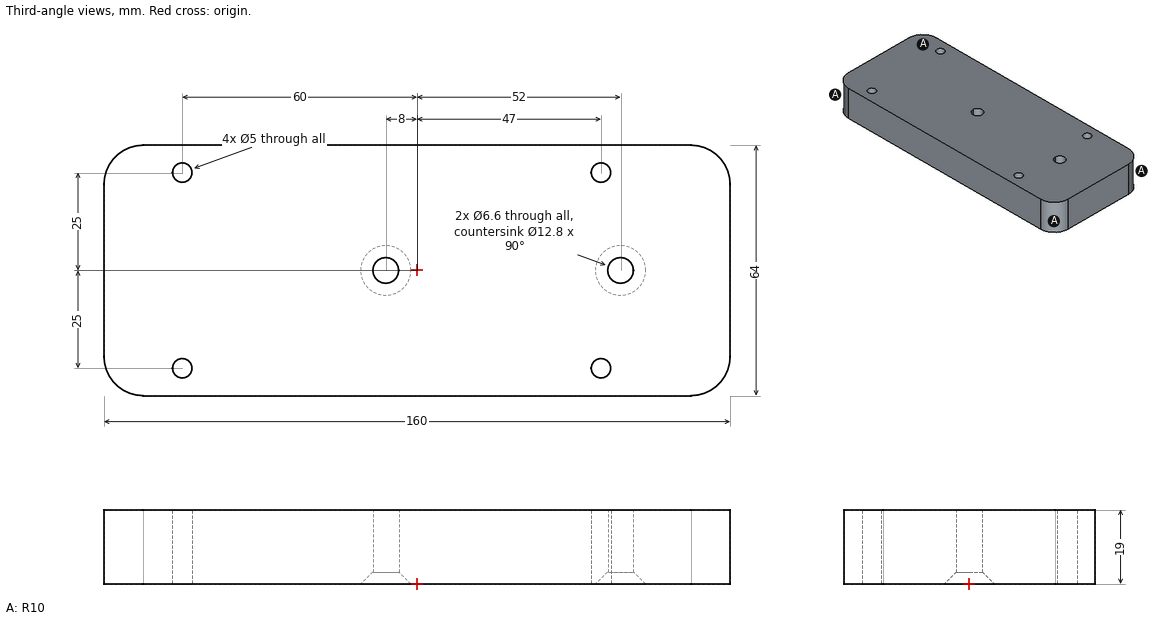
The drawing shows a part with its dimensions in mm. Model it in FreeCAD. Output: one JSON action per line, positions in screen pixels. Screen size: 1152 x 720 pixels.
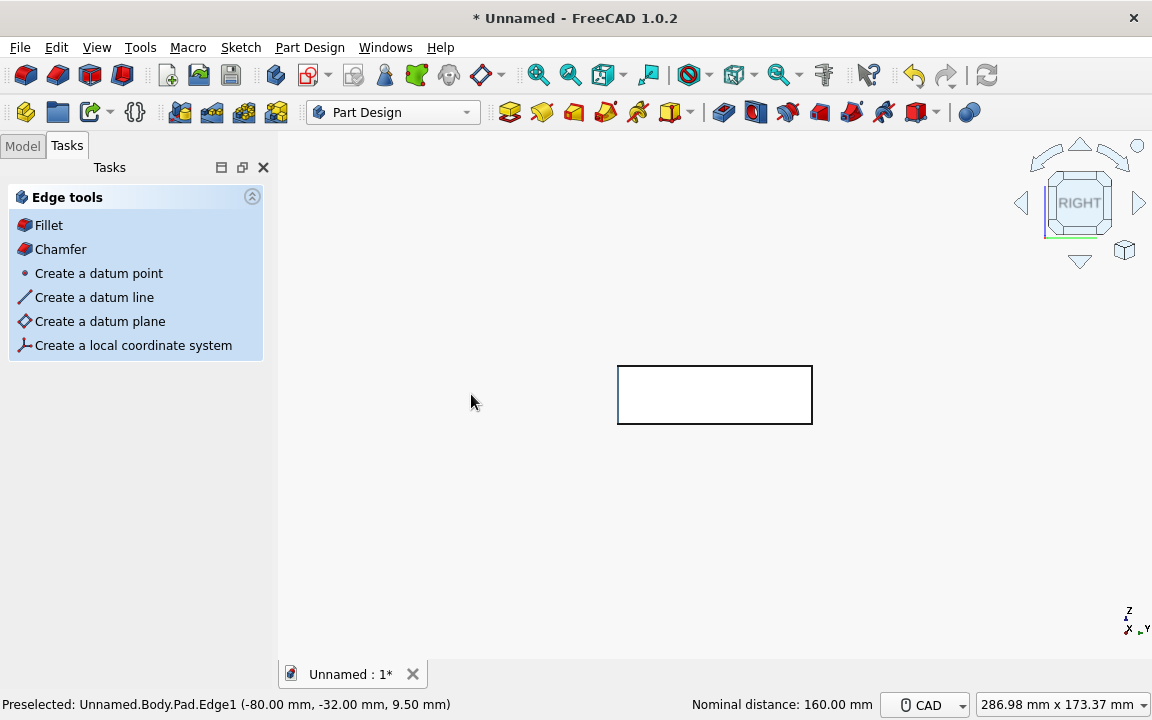
{"action": "left_click", "coordinate": [540, 76]}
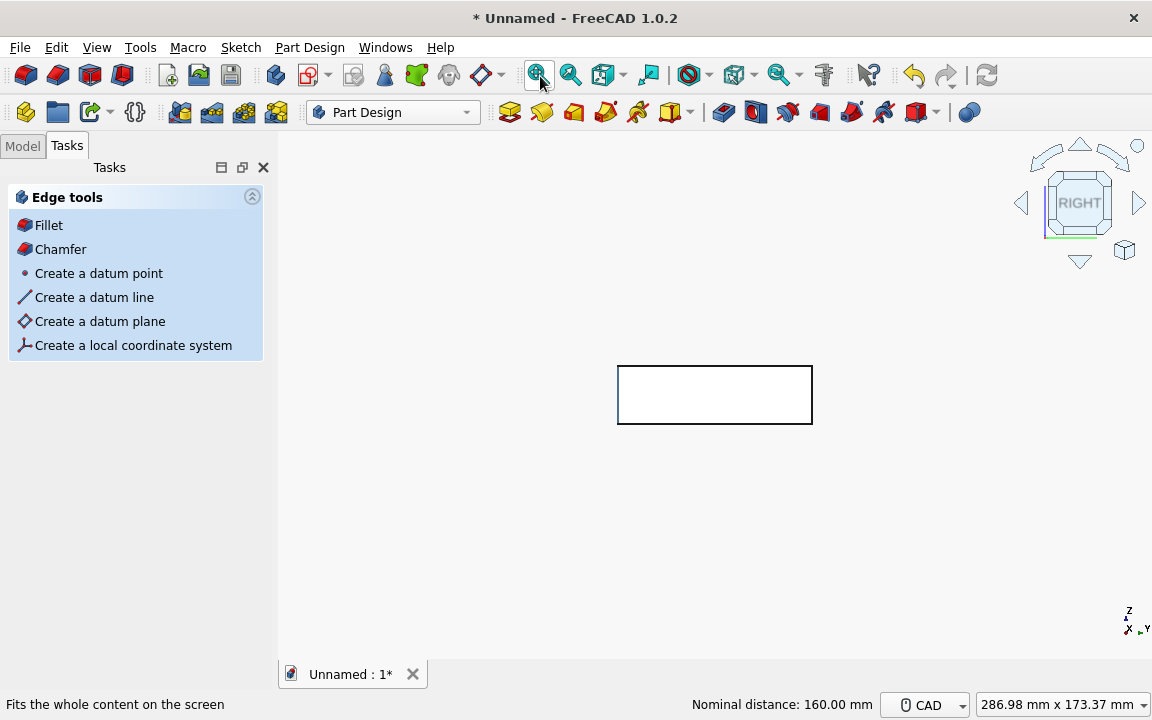
{"action": "left_click", "coordinate": [812, 394], "text": "ctrl"}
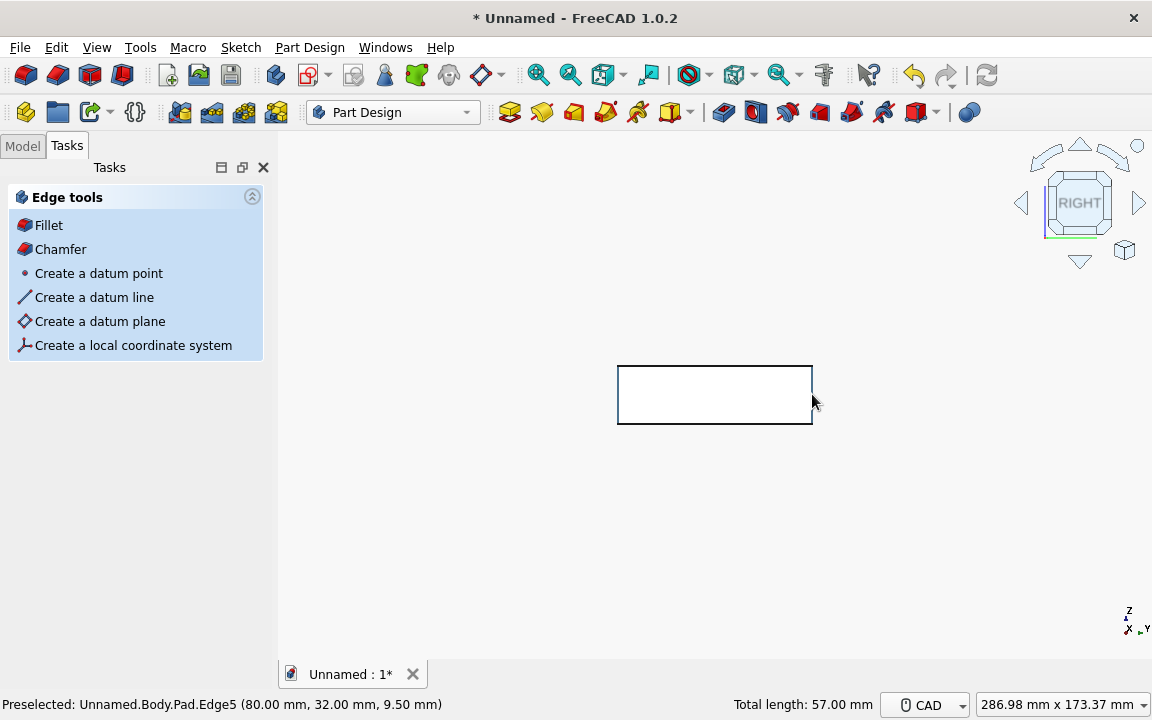
{"action": "key", "text": "5"}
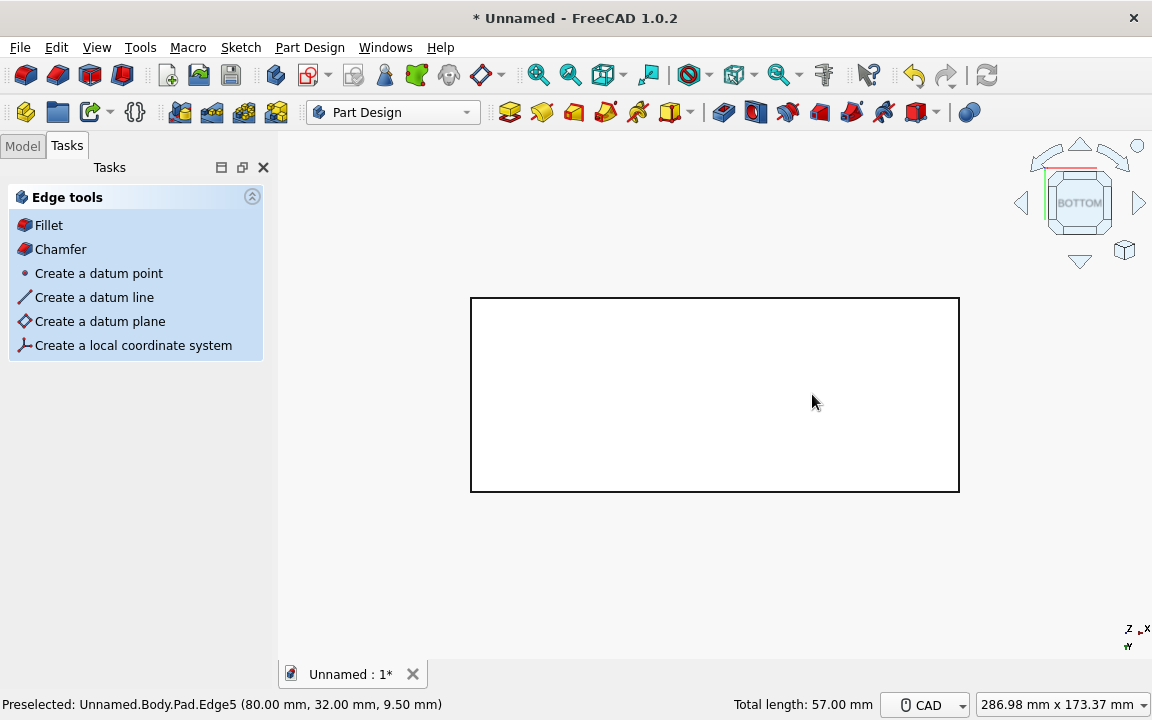
{"action": "key", "text": "4"}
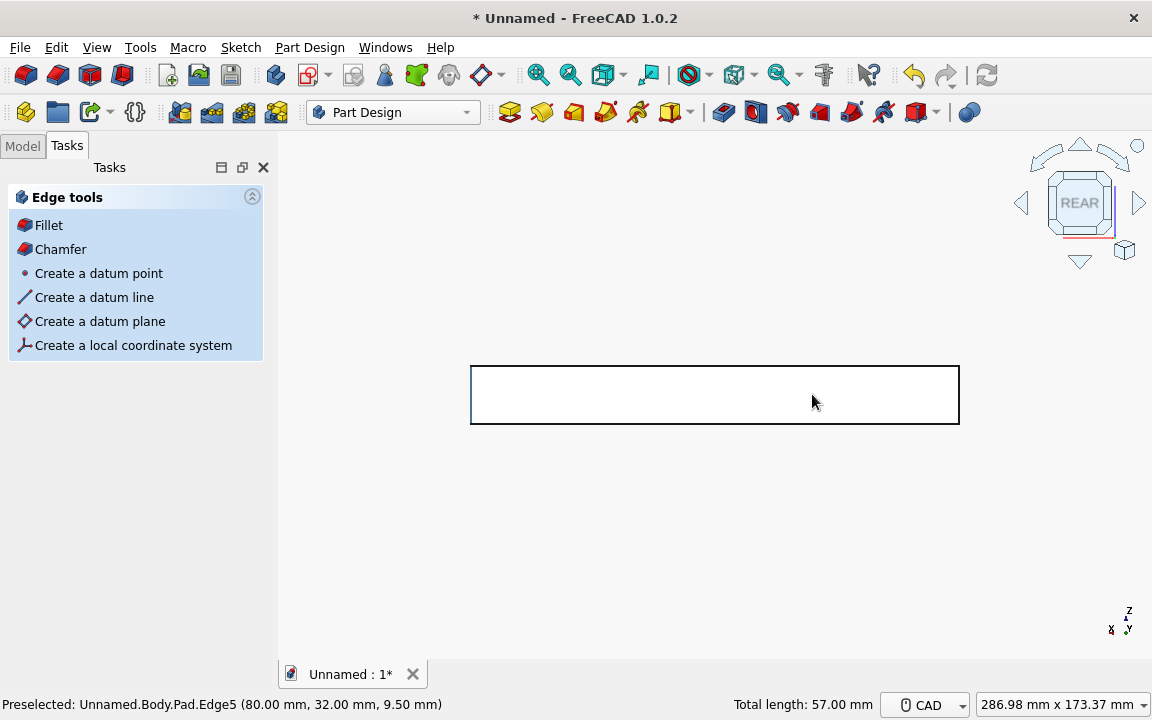
{"action": "left_click", "coordinate": [959, 394], "text": "ctrl"}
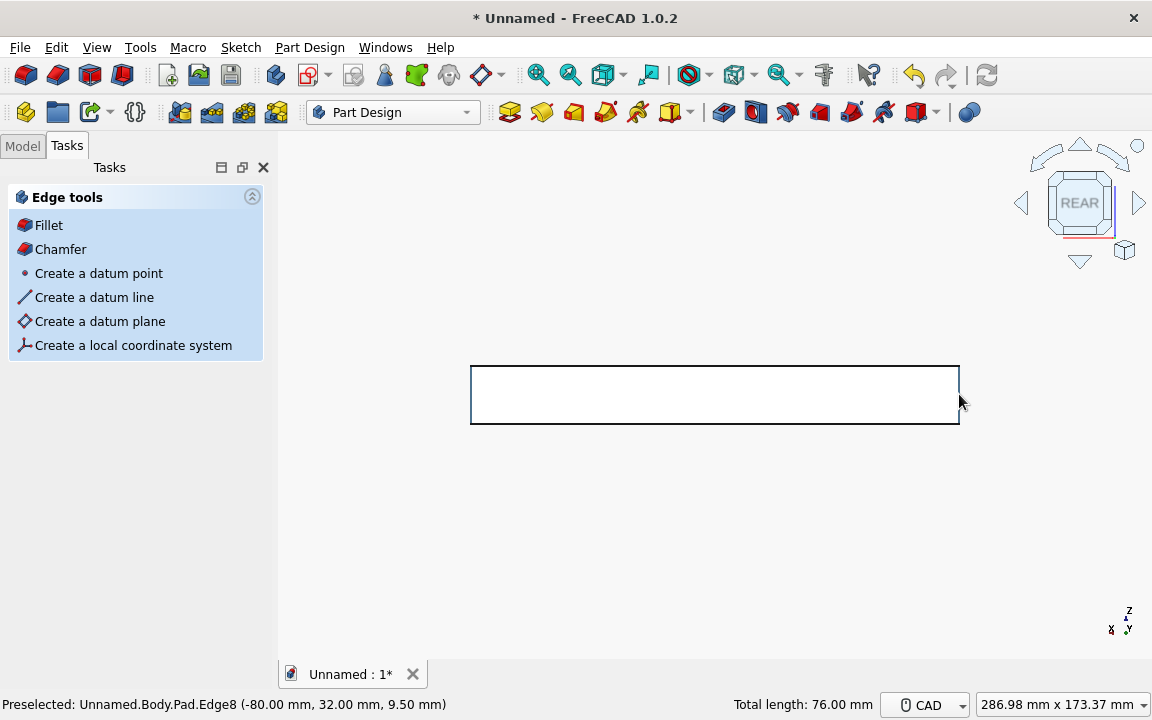
{"action": "left_click", "coordinate": [26, 76]}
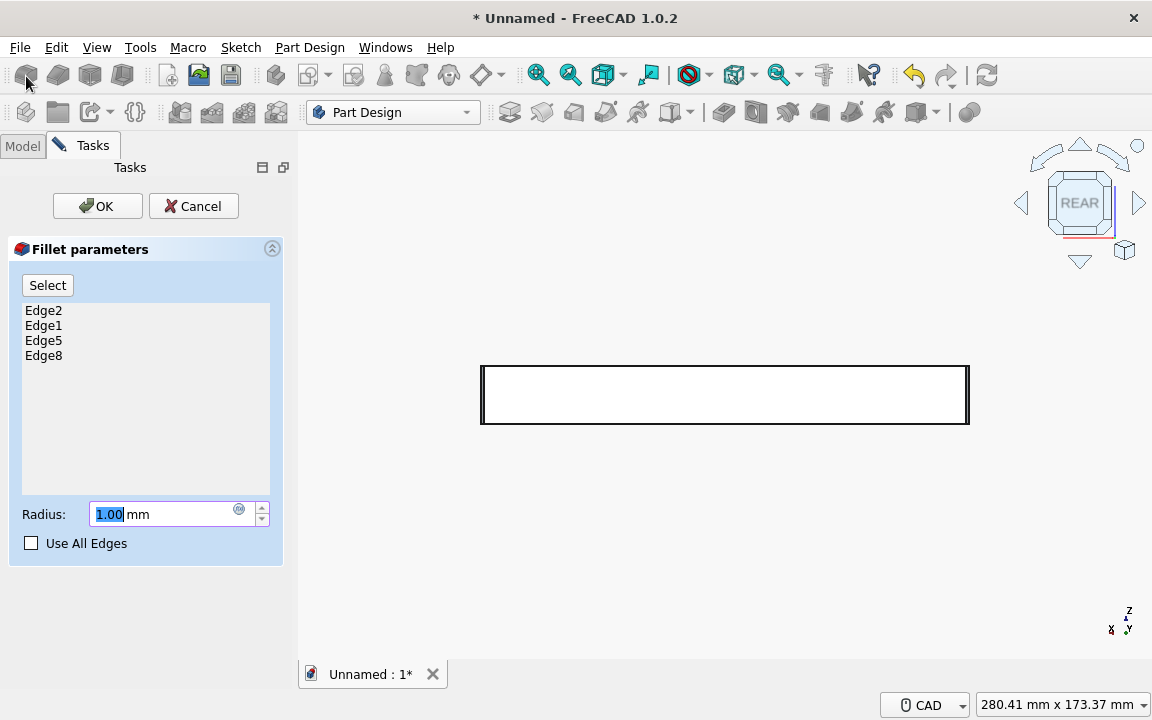
{"action": "type", "text": "10"}
{"action": "key", "text": "Tab"}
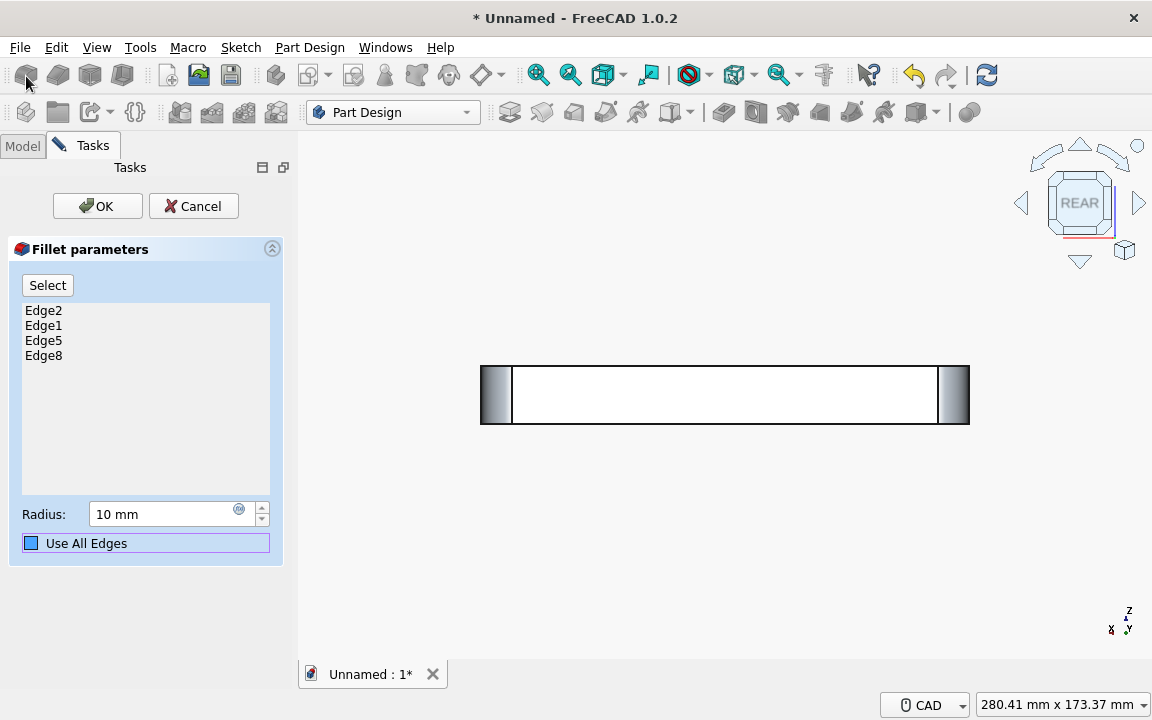
{"action": "left_click", "coordinate": [98, 206]}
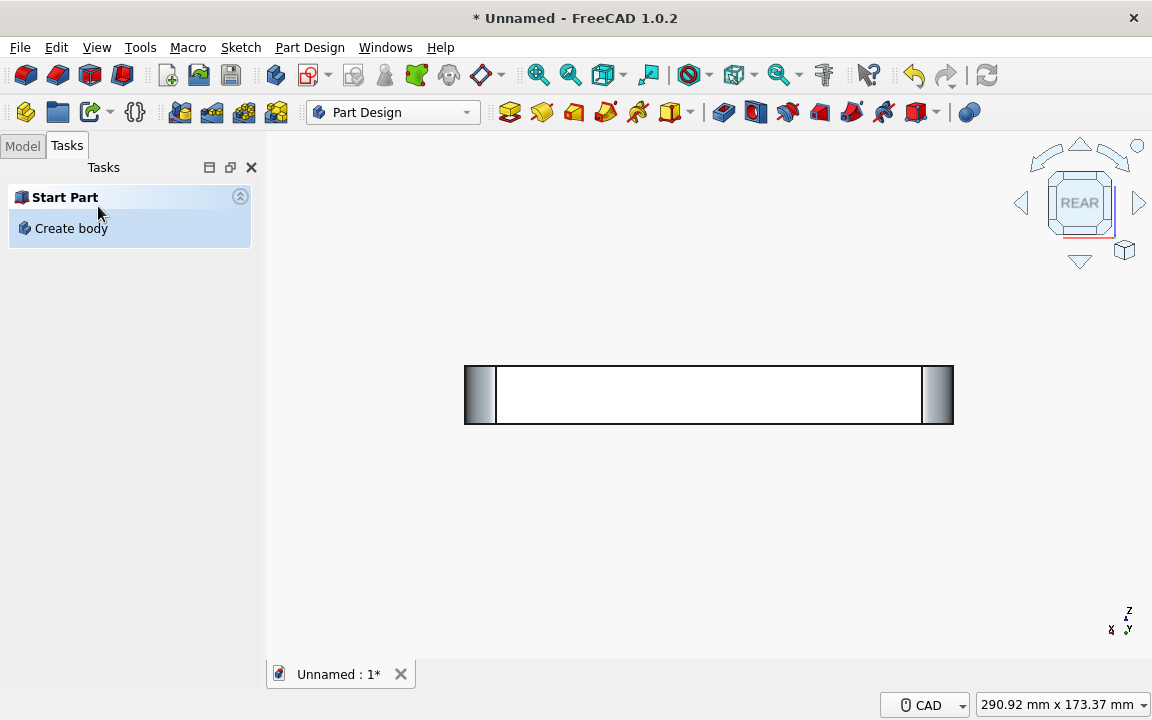
{"action": "key", "text": "0"}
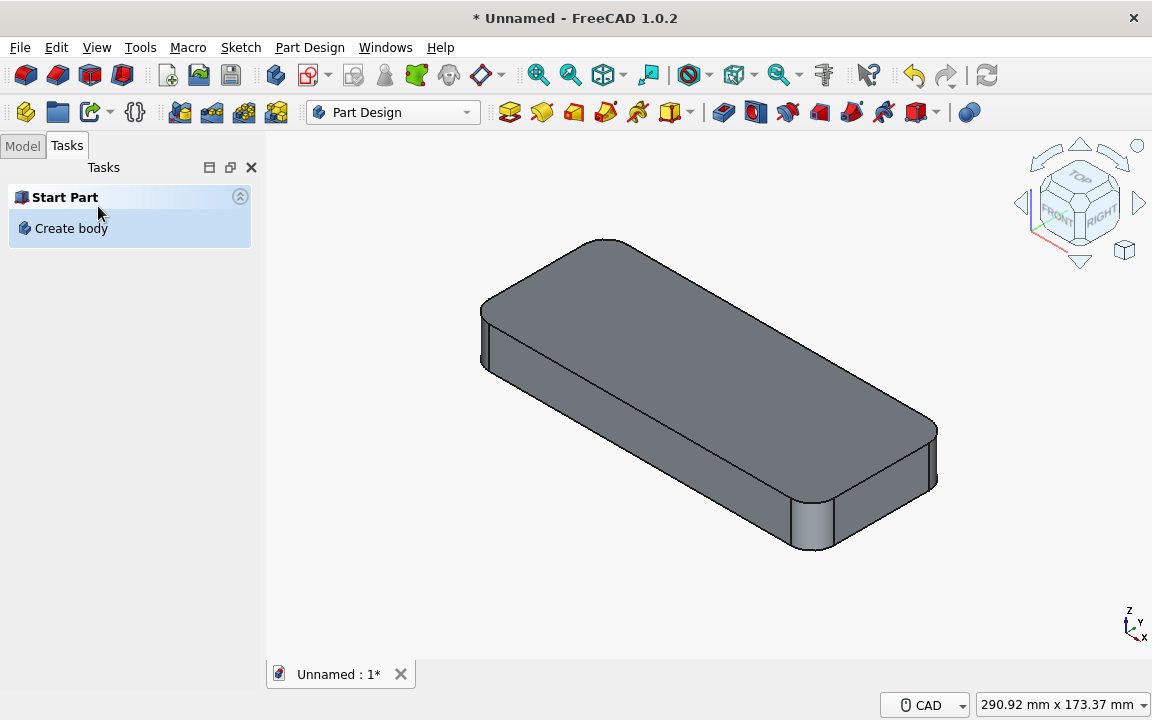
{"action": "left_click", "coordinate": [807, 427]}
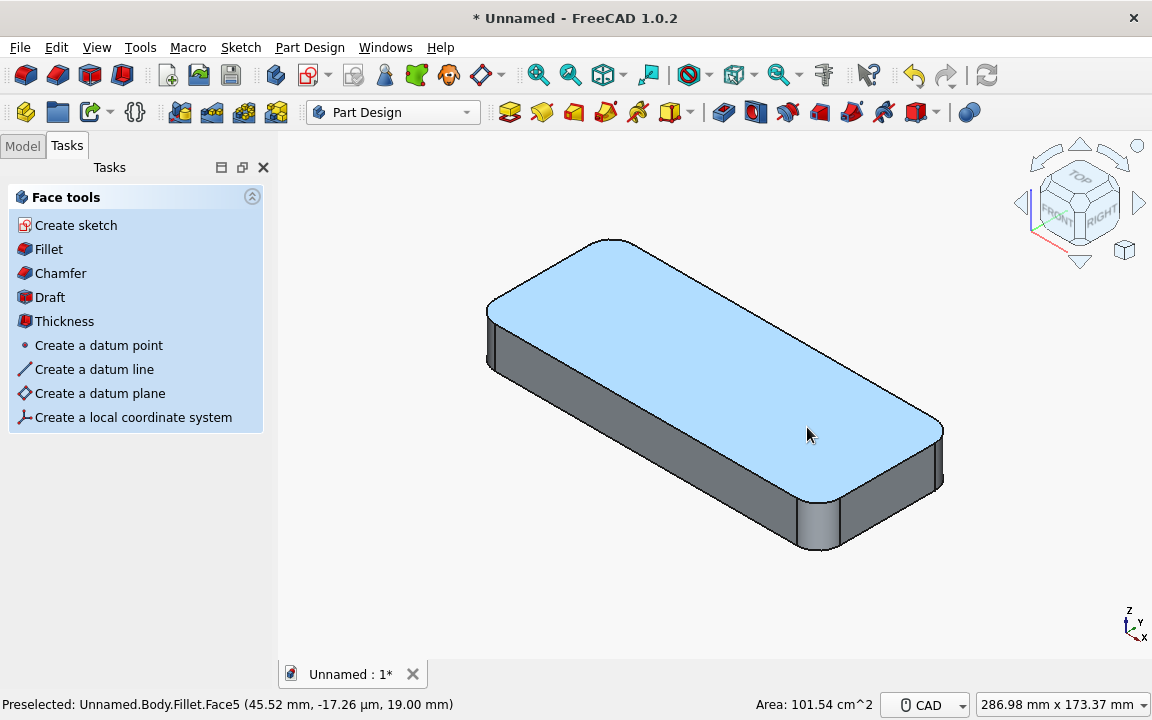
{"action": "left_click", "coordinate": [308, 76]}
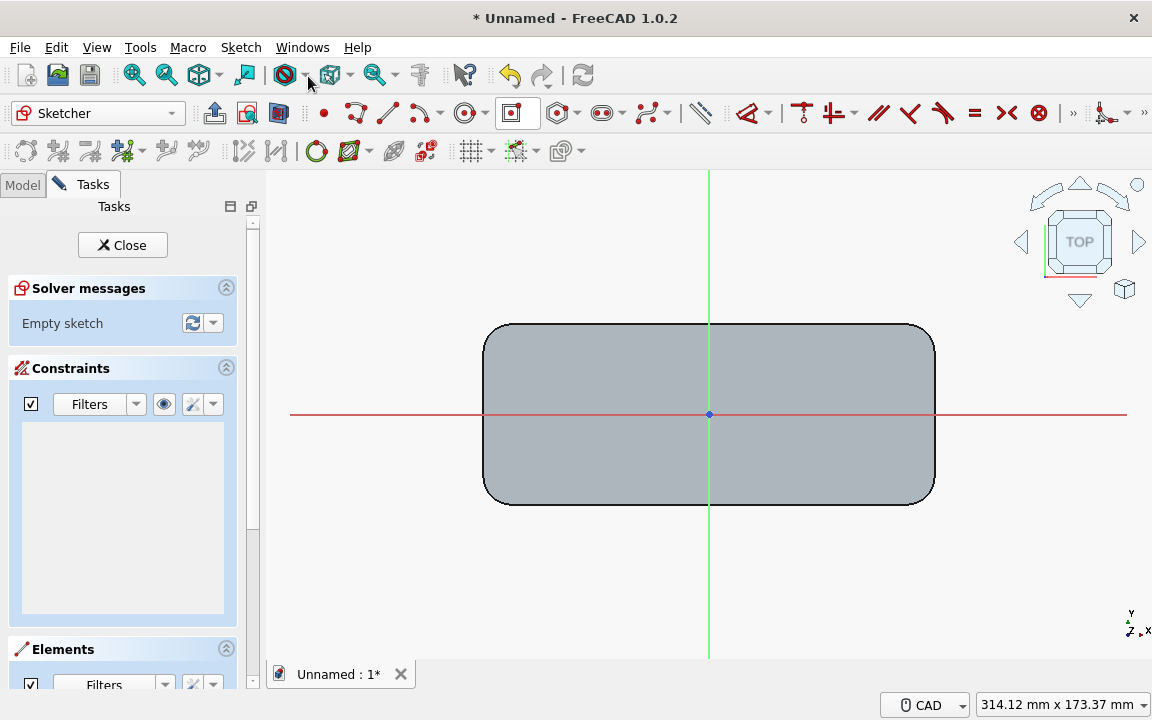
{"action": "scroll", "coordinate": [793, 415], "scroll_direction": "up", "scroll_amount": 2}